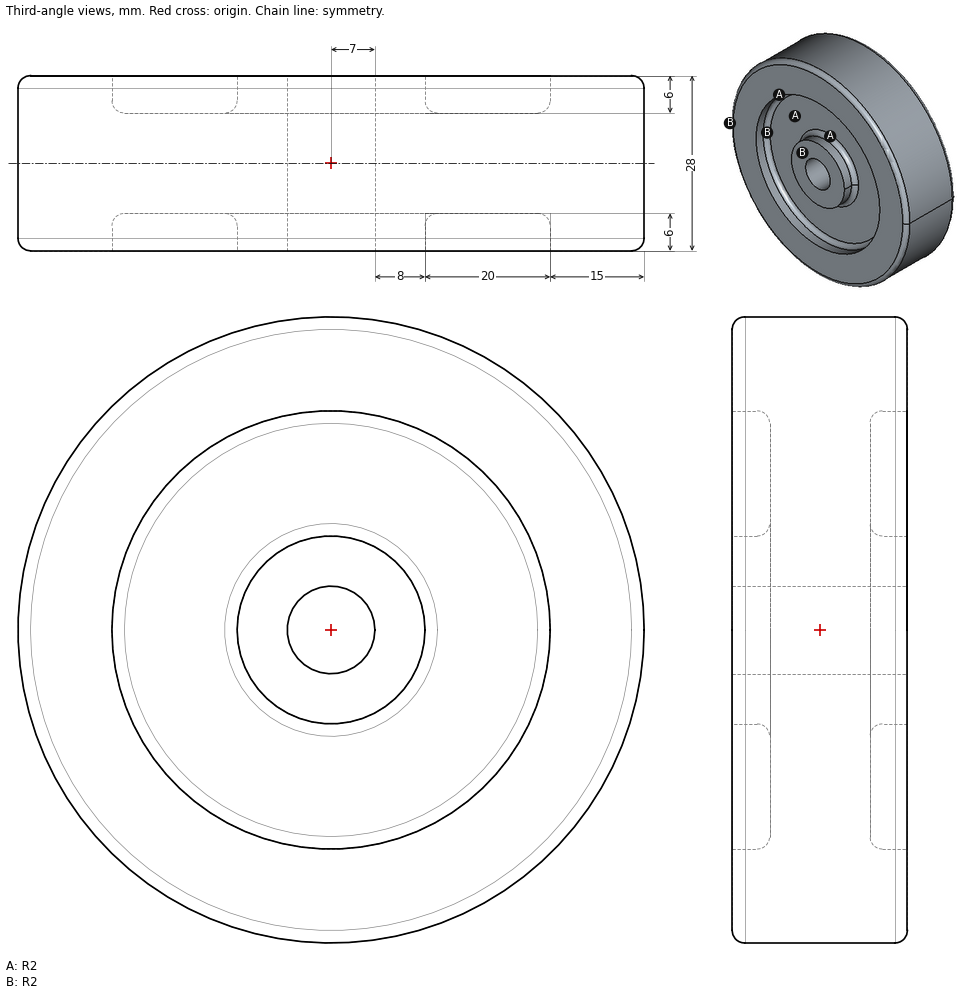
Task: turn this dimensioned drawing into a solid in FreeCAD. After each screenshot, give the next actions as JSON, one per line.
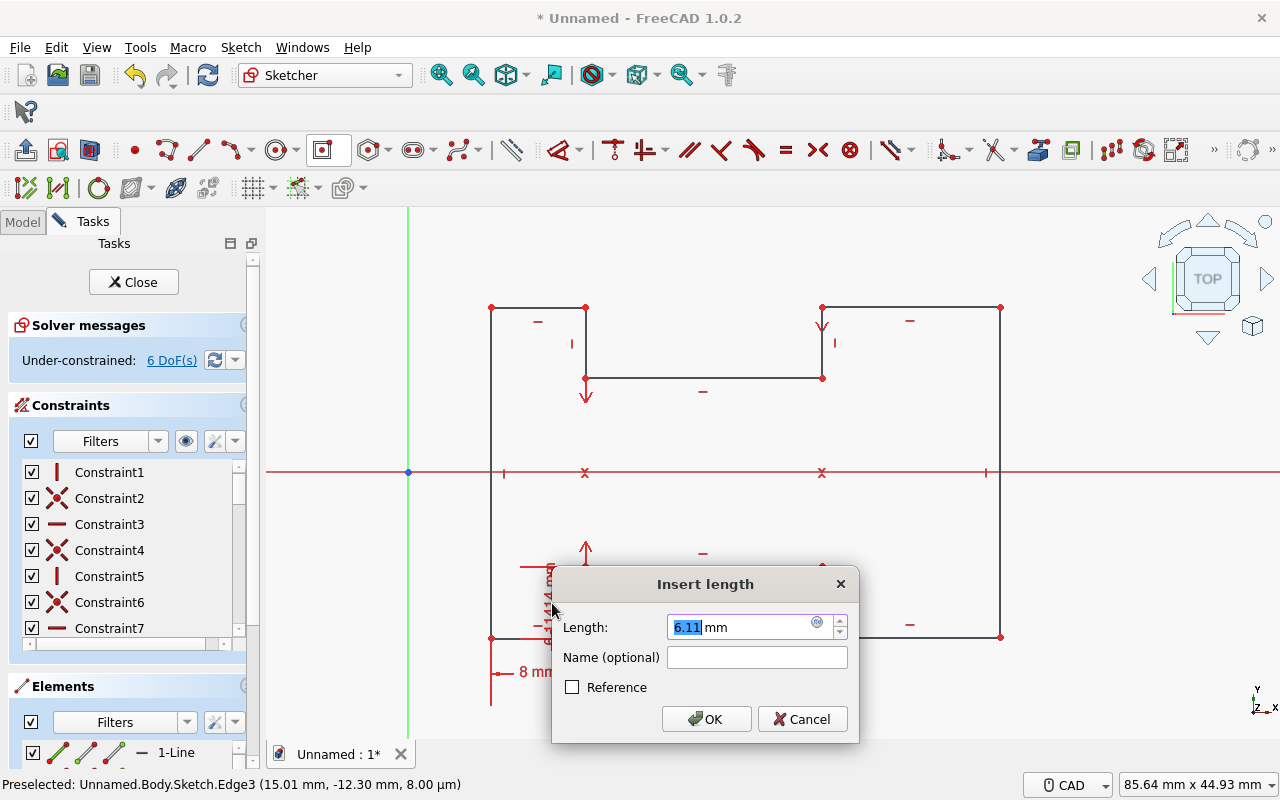
{"action": "type", "text": "6"}
{"action": "key", "text": "Return"}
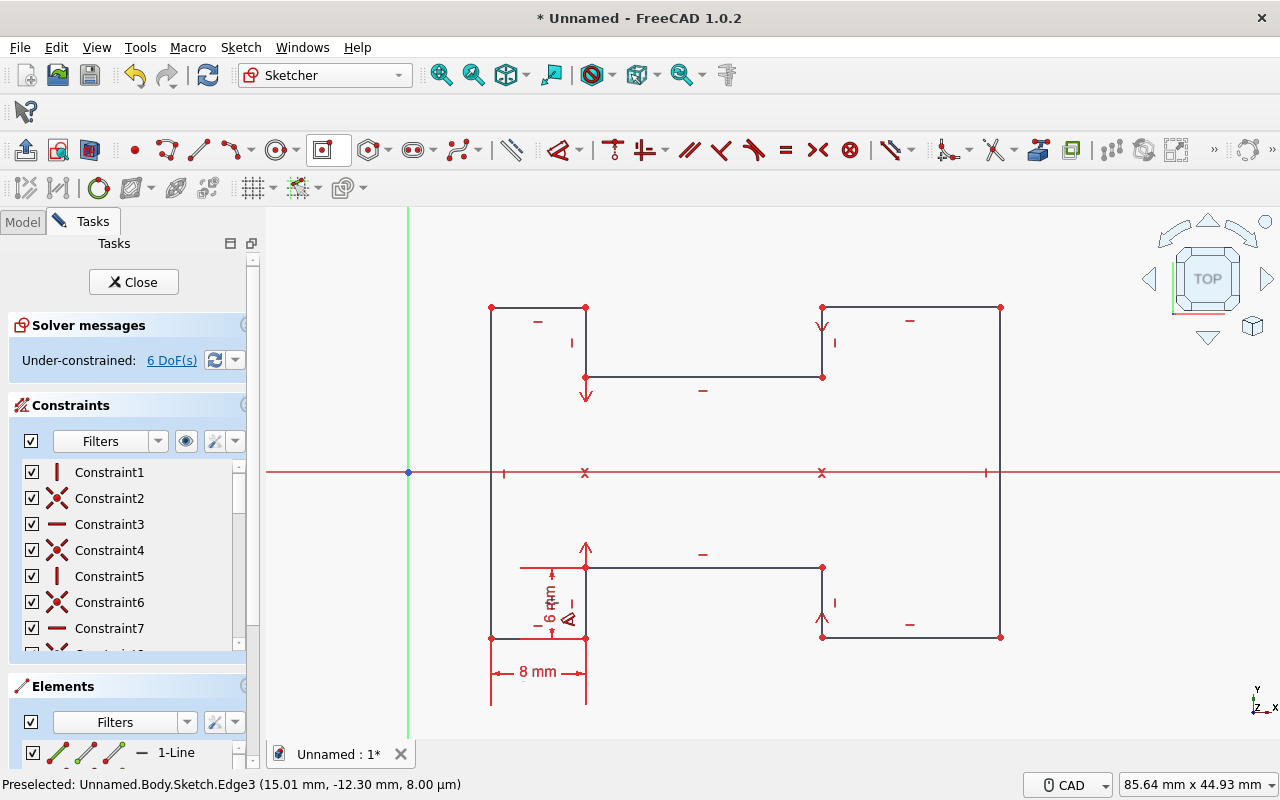
{"action": "left_click", "coordinate": [822, 589]}
{"action": "left_click", "coordinate": [856, 603]}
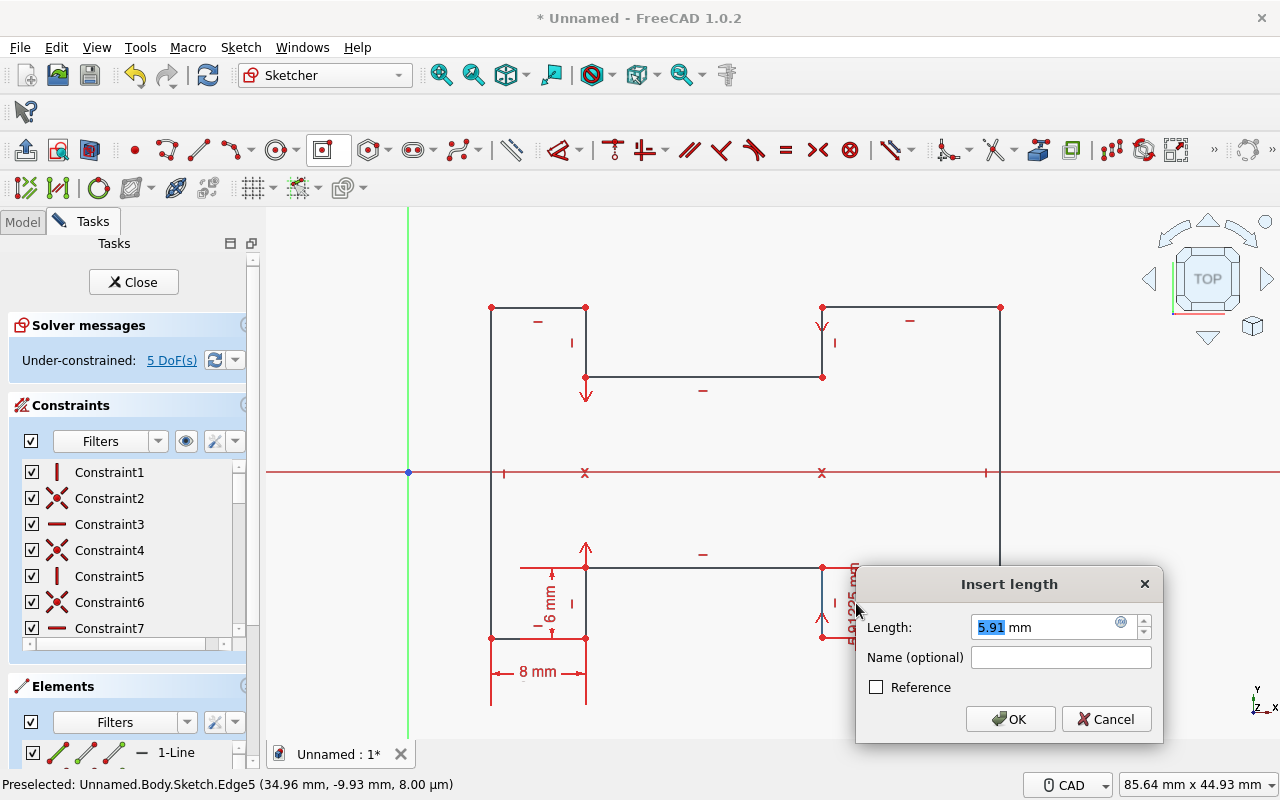
{"action": "type", "text": "6"}
{"action": "key", "text": "Return"}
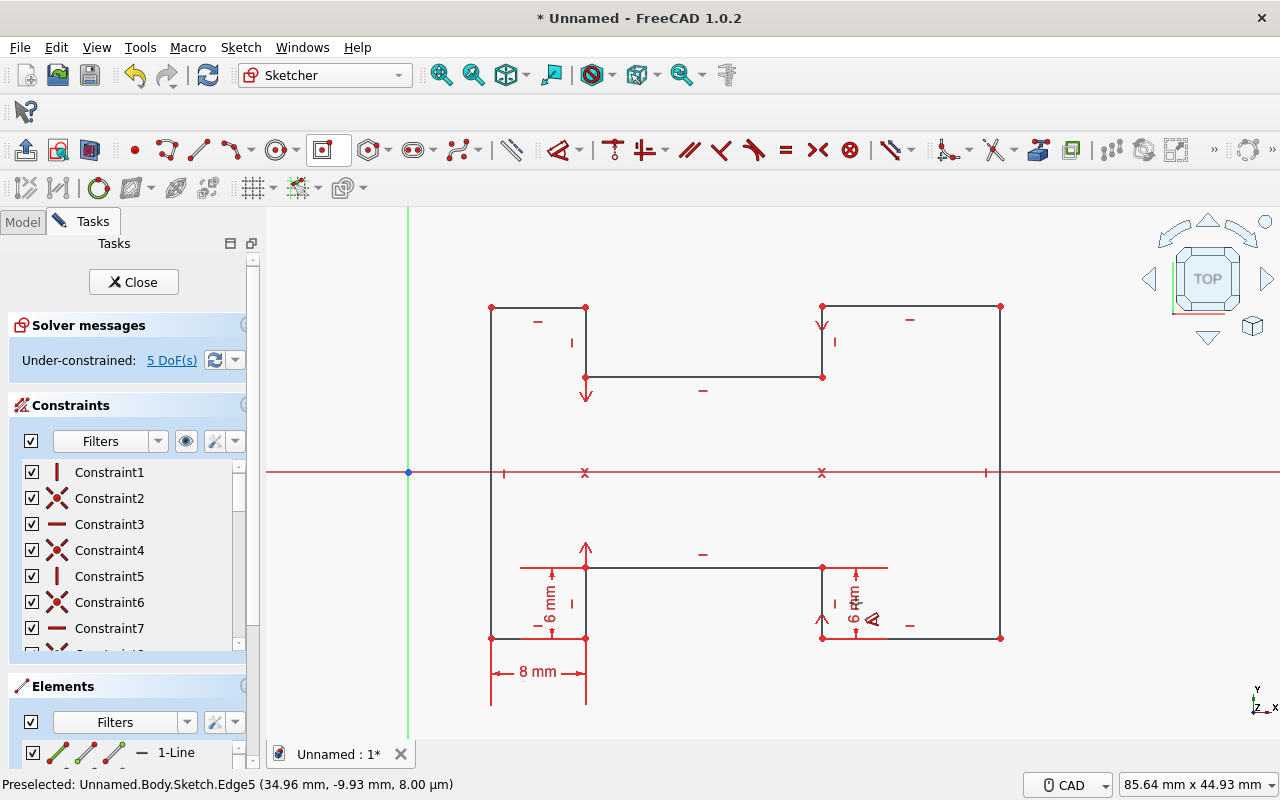
{"action": "left_click", "coordinate": [586, 356]}
{"action": "left_click", "coordinate": [552, 343]}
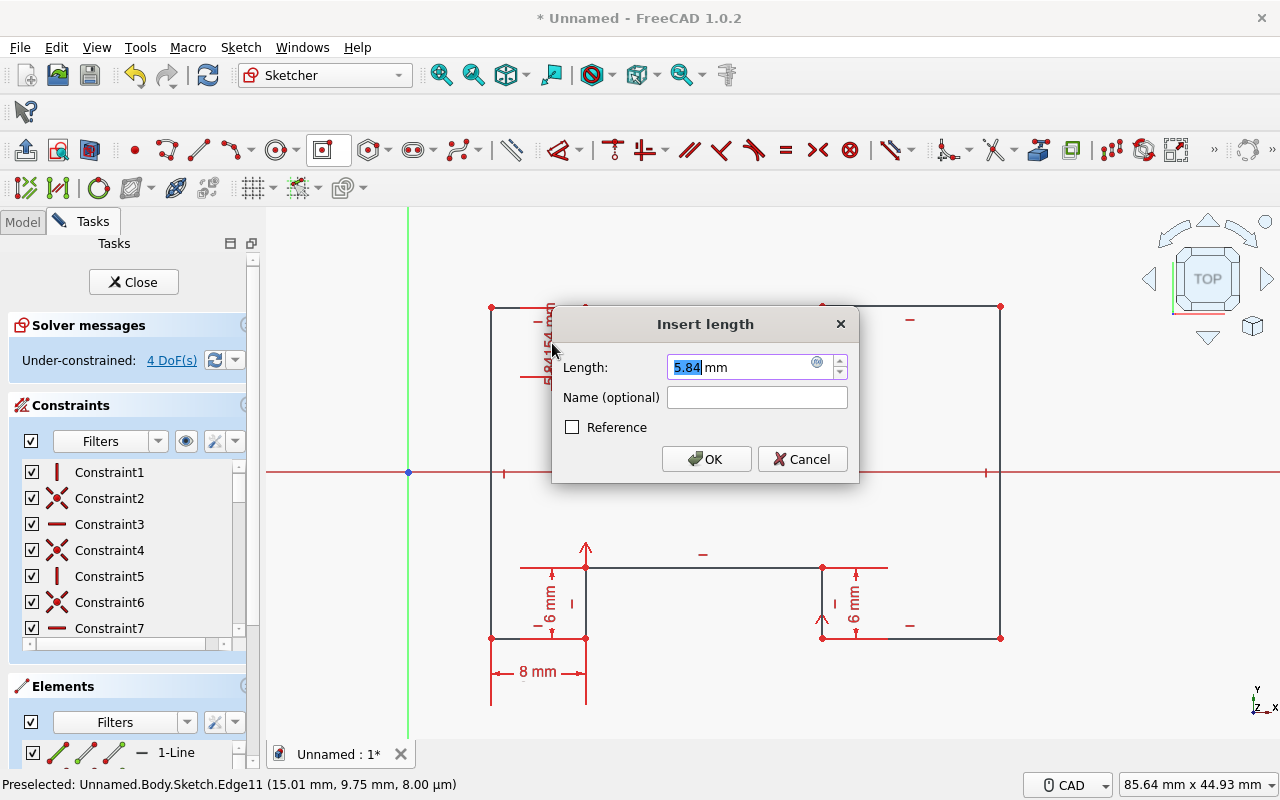
{"action": "type", "text": "6"}
{"action": "key", "text": "Return"}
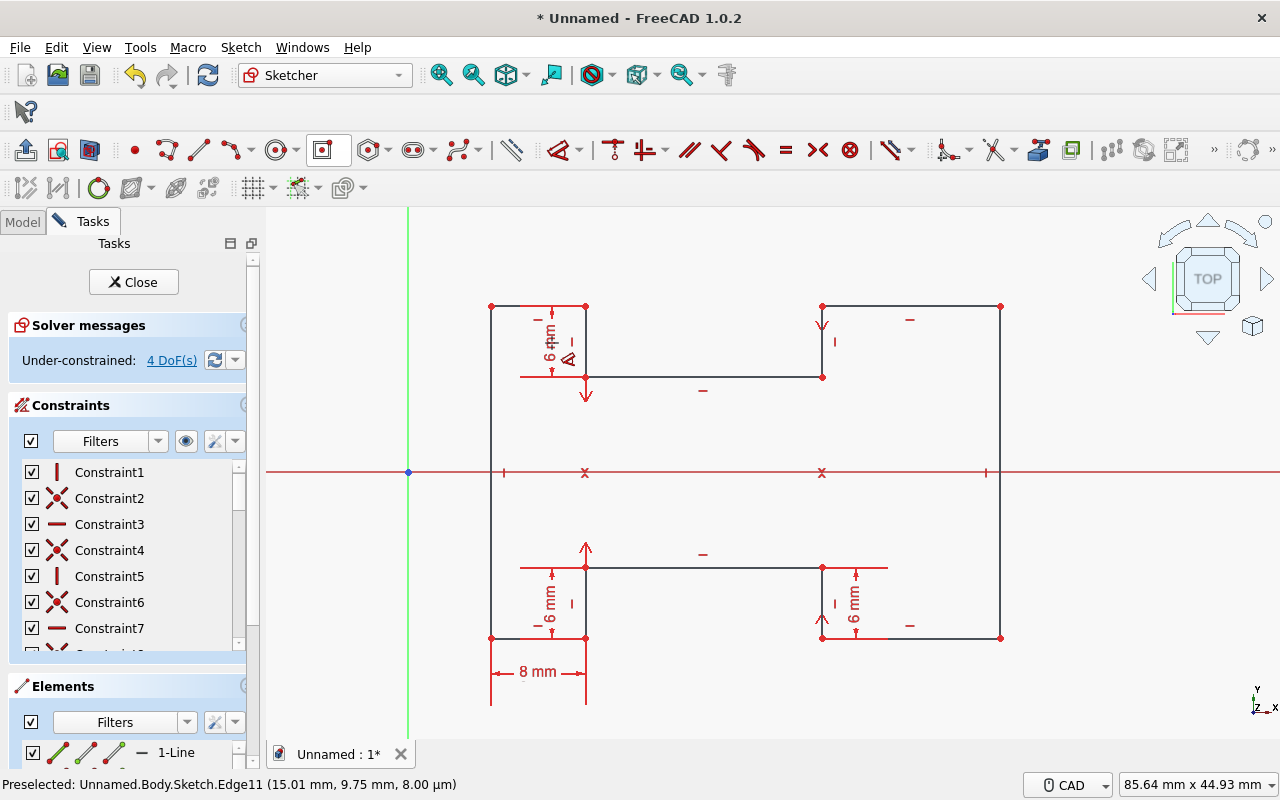
{"action": "left_click", "coordinate": [491, 406]}
{"action": "left_click", "coordinate": [457, 396]}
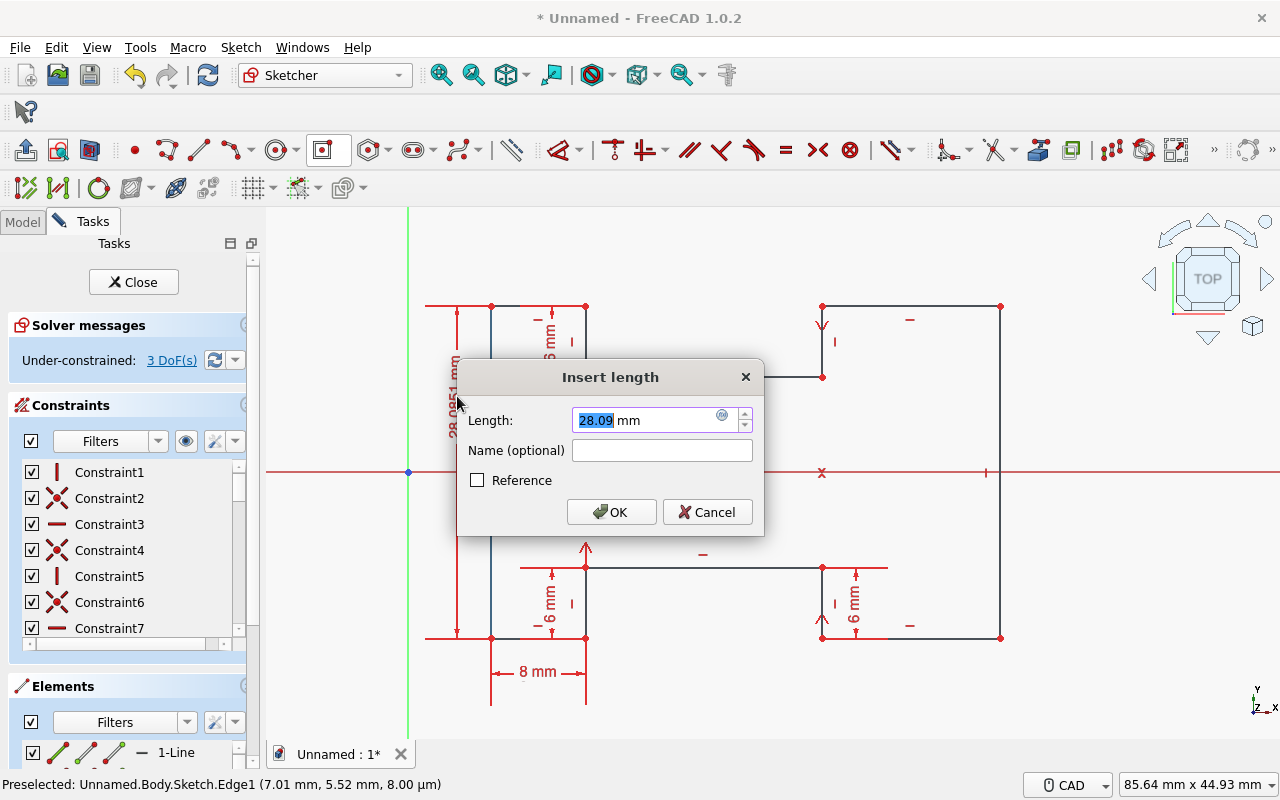
{"action": "type", "text": "28"}
{"action": "key", "text": "Return"}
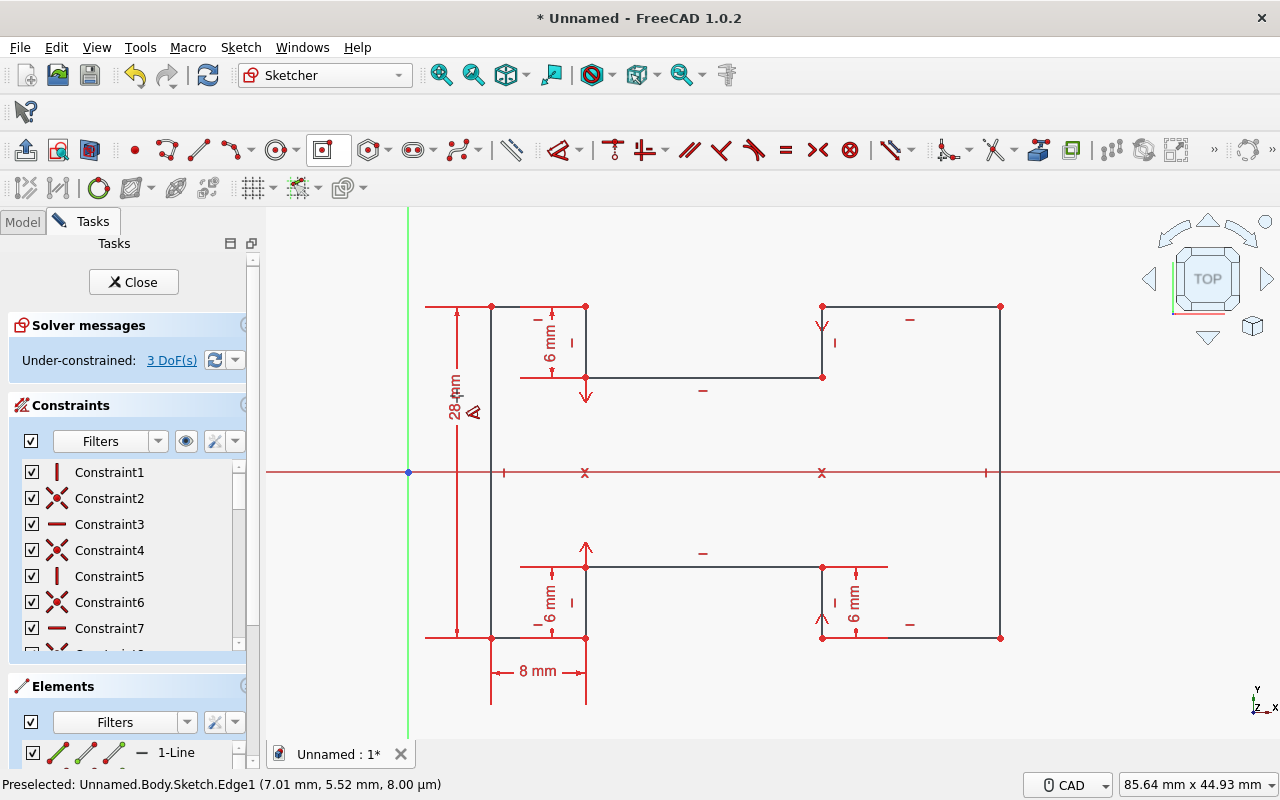
{"action": "left_click", "coordinate": [657, 567]}
{"action": "left_click", "coordinate": [704, 601]}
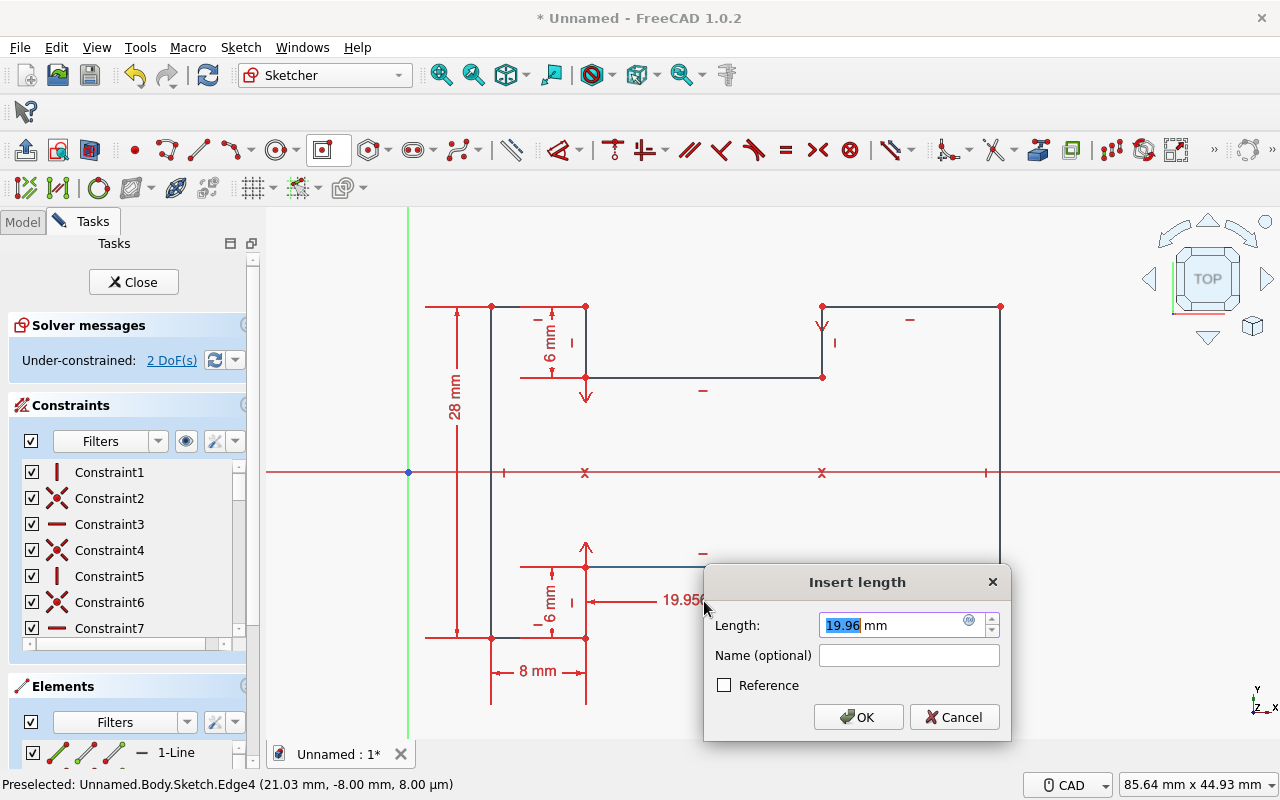
{"action": "type", "text": "20"}
{"action": "key", "text": "Return"}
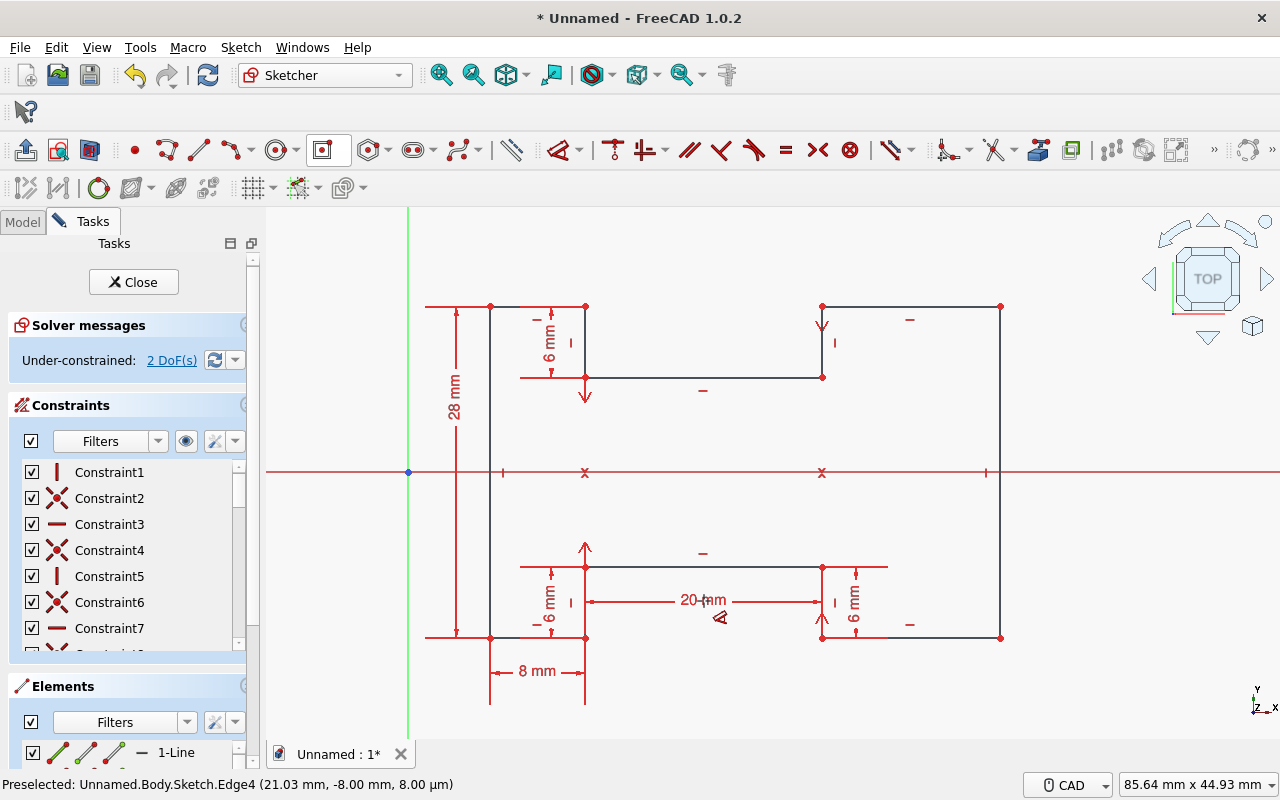
{"action": "left_click", "coordinate": [875, 638]}
{"action": "left_click", "coordinate": [911, 672]}